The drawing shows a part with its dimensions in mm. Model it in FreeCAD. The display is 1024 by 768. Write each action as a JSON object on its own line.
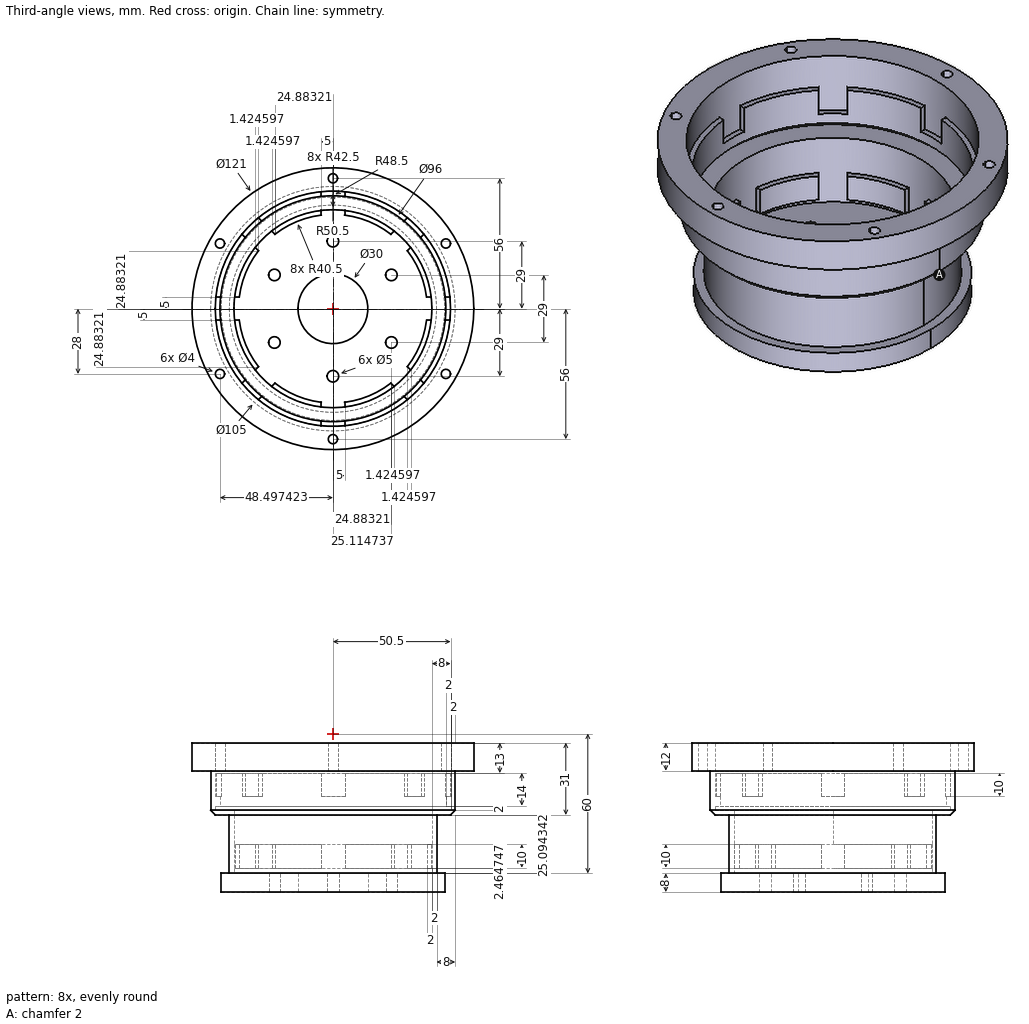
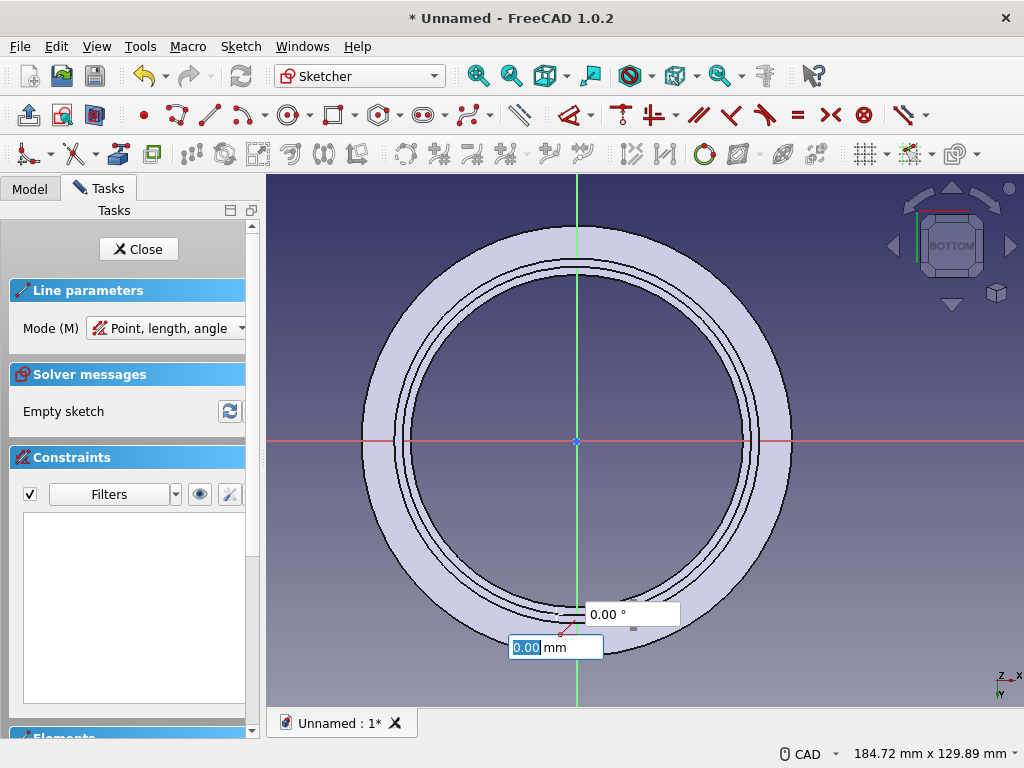
{"action": "scroll", "coordinate": [556, 606], "scroll_direction": "up", "scroll_amount": 4}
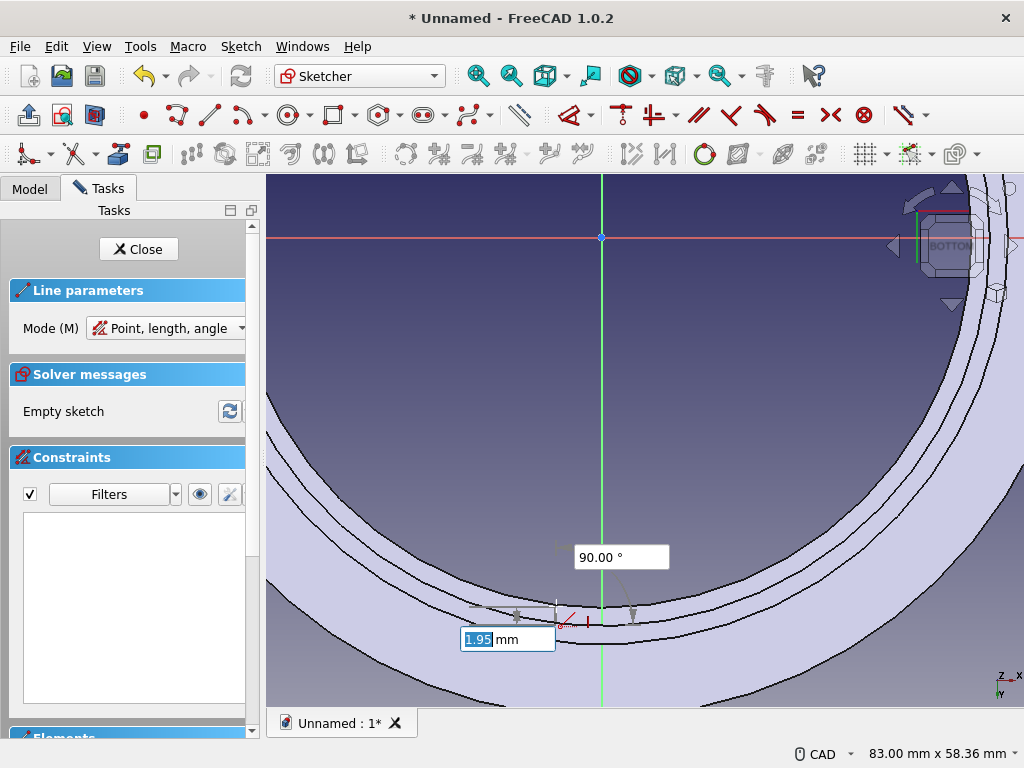
{"action": "left_click", "coordinate": [556, 605]}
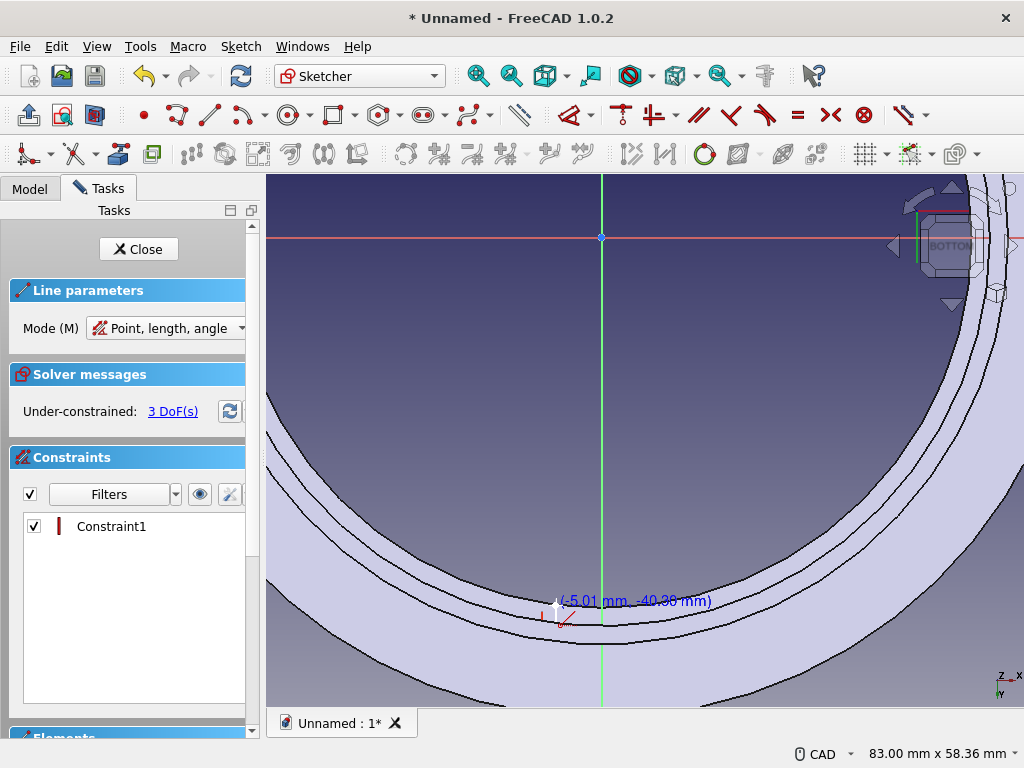
{"action": "left_click", "coordinate": [374, 530]}
{"action": "left_click", "coordinate": [361, 543]}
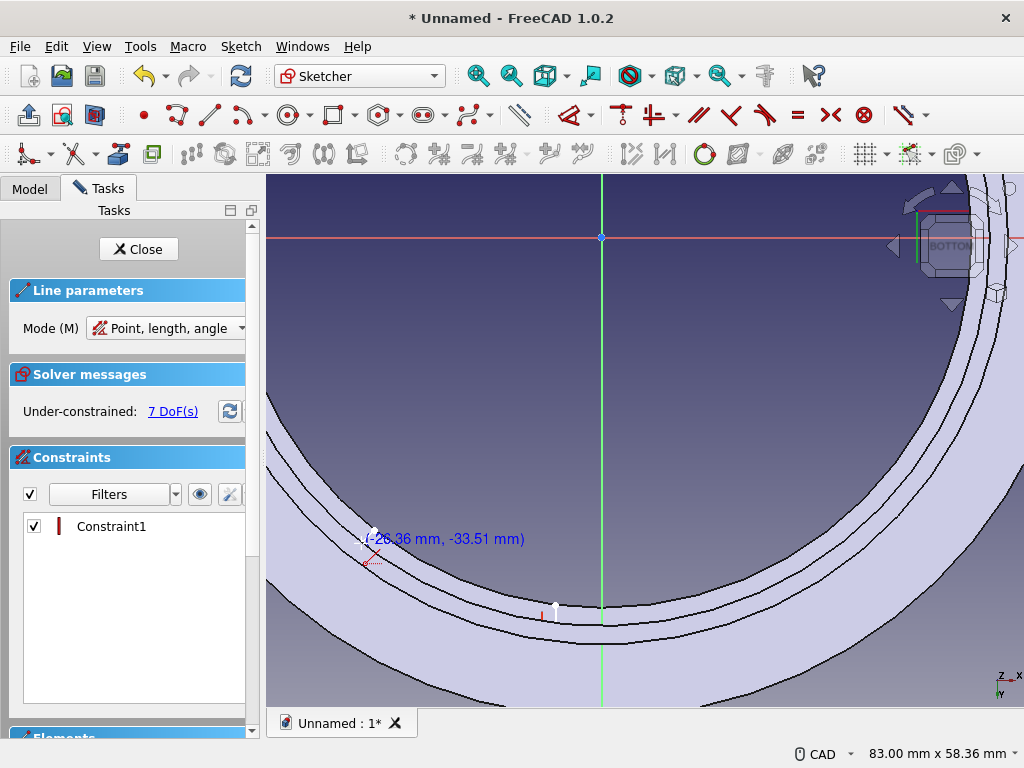
{"action": "left_click", "coordinate": [297, 478]}
{"action": "left_click", "coordinate": [310, 465]}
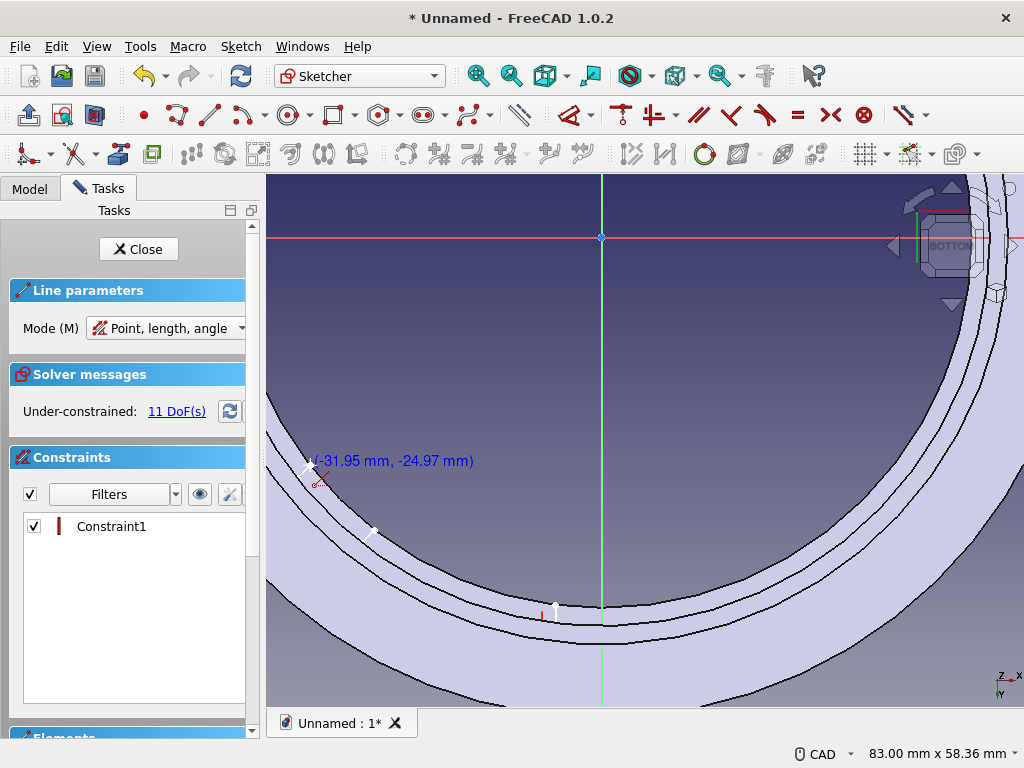
{"action": "scroll", "coordinate": [556, 606], "scroll_direction": "down", "scroll_amount": 4}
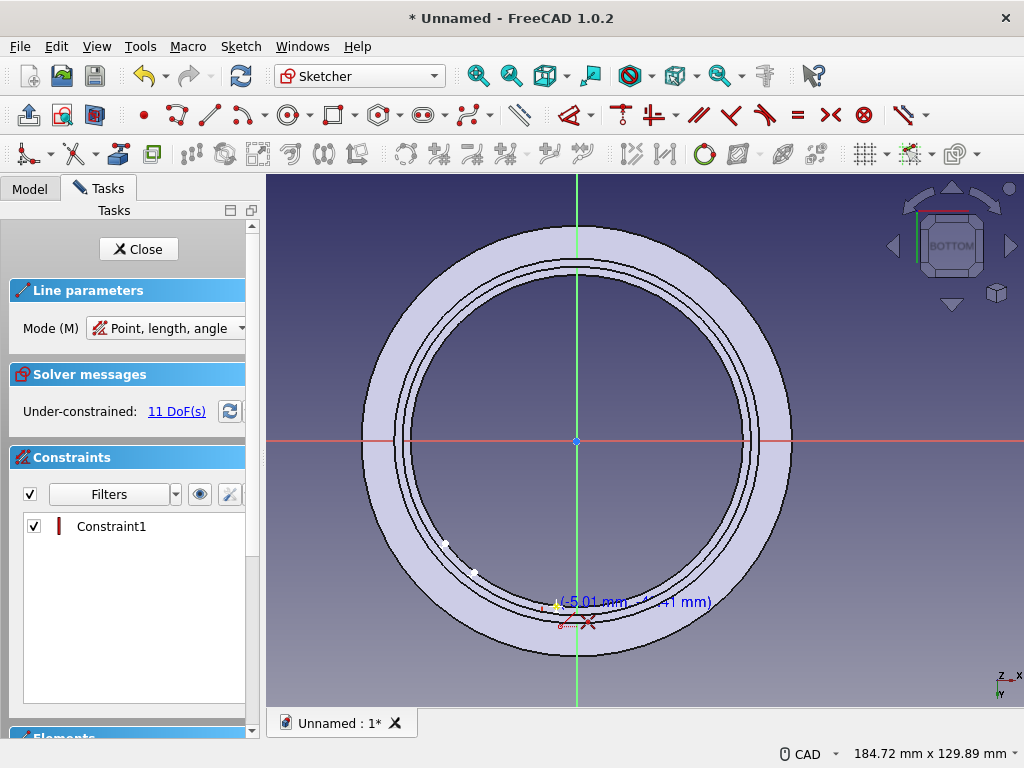
{"action": "left_click", "coordinate": [412, 462]}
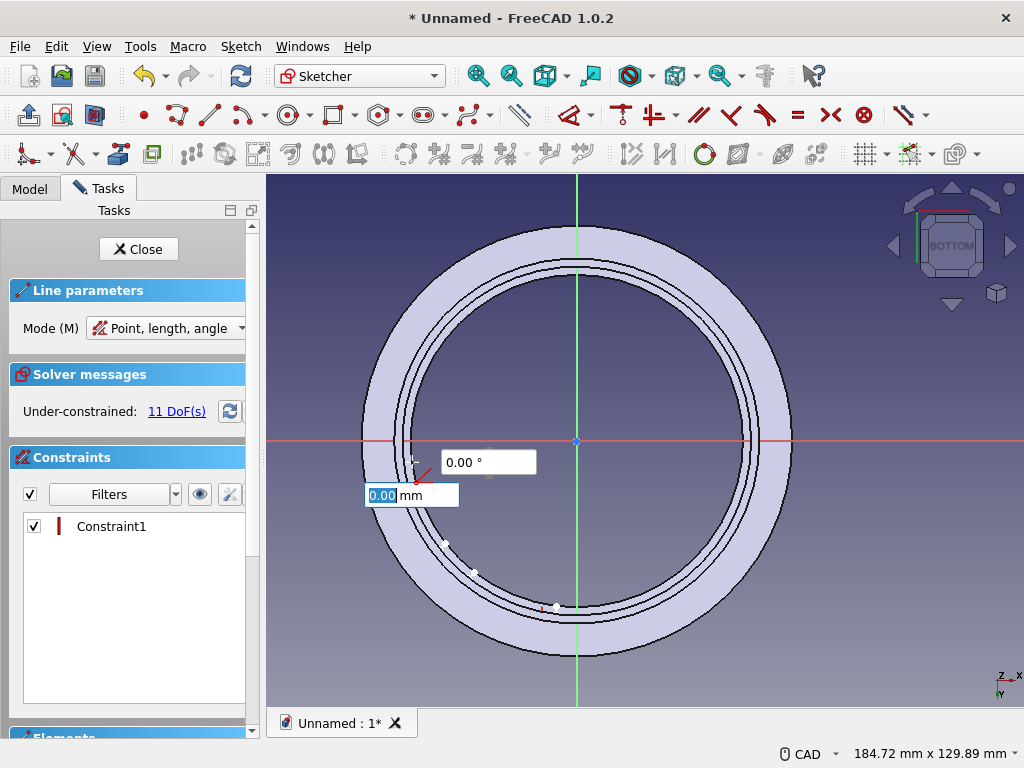
{"action": "scroll", "coordinate": [404, 462], "scroll_direction": "up", "scroll_amount": 4}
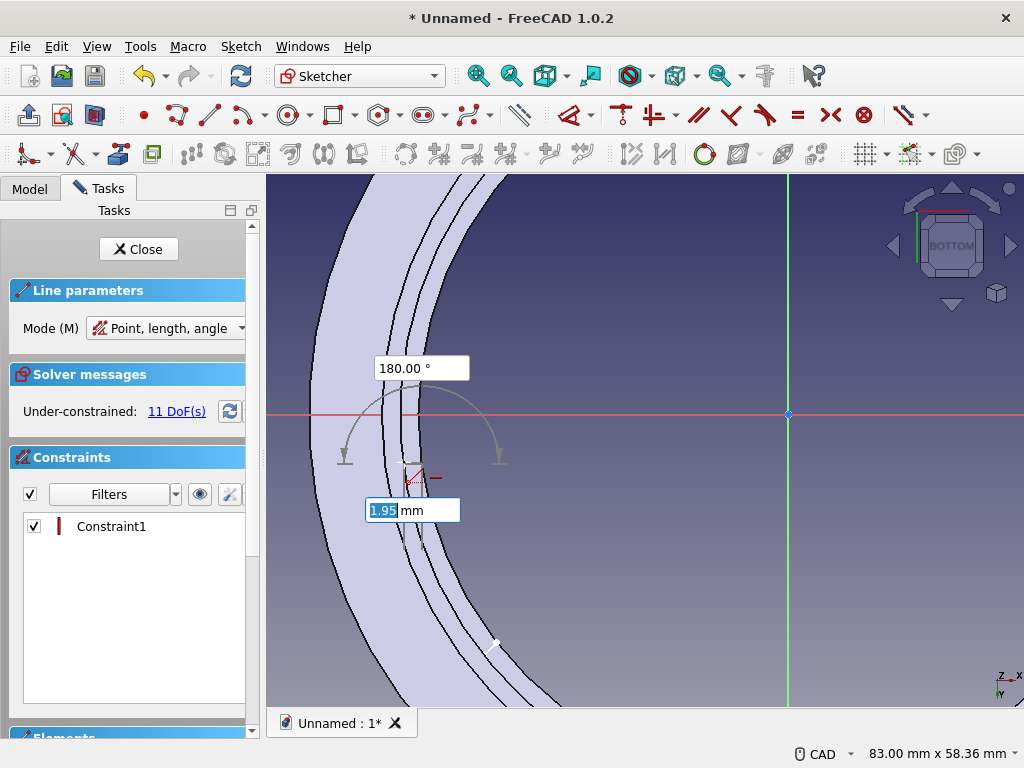
{"action": "left_click", "coordinate": [403, 461]}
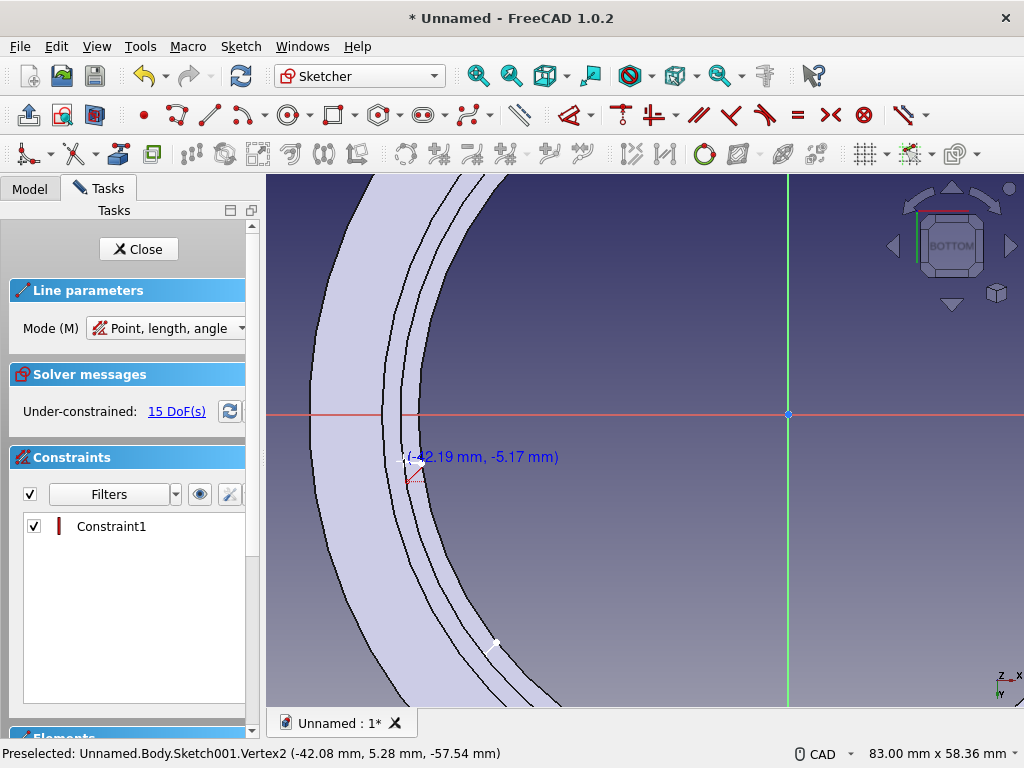
{"action": "left_click", "coordinate": [403, 369]}
{"action": "left_click", "coordinate": [421, 369]}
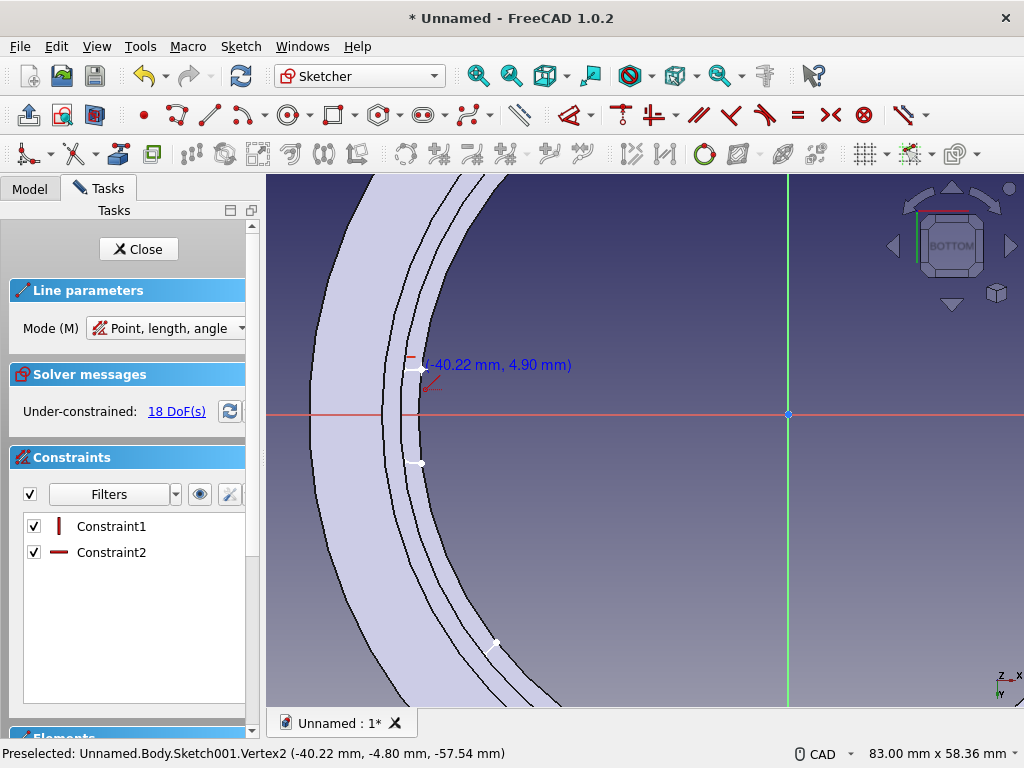
{"action": "scroll", "coordinate": [404, 462], "scroll_direction": "down", "scroll_amount": 4}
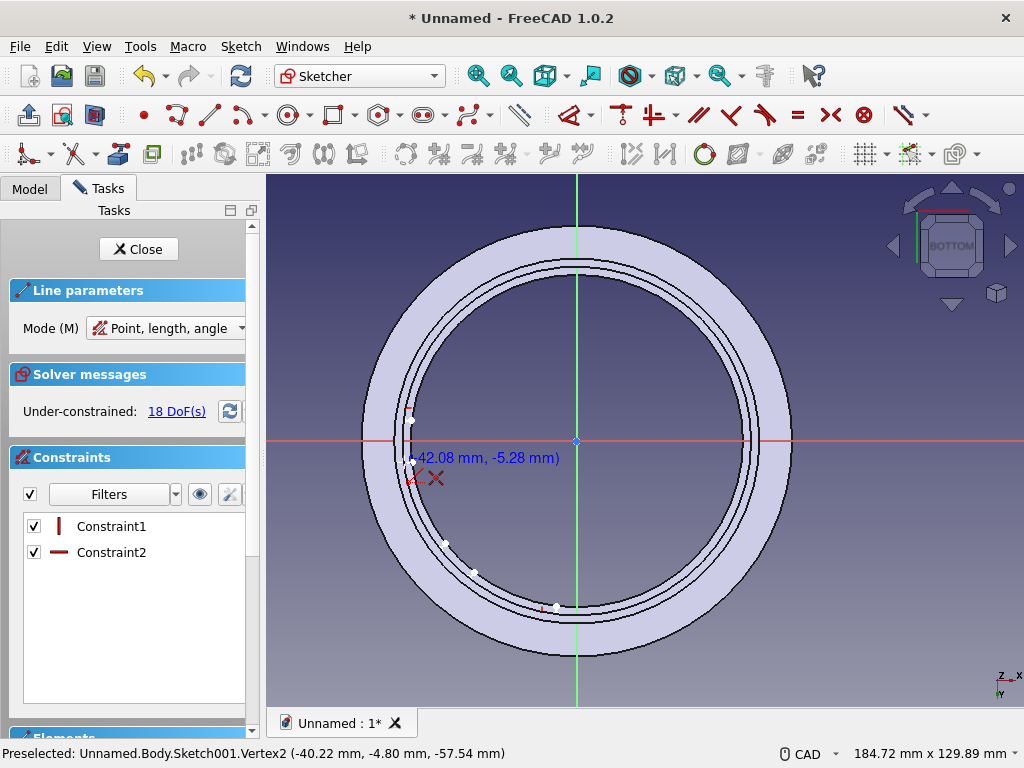
{"action": "left_click", "coordinate": [446, 339]}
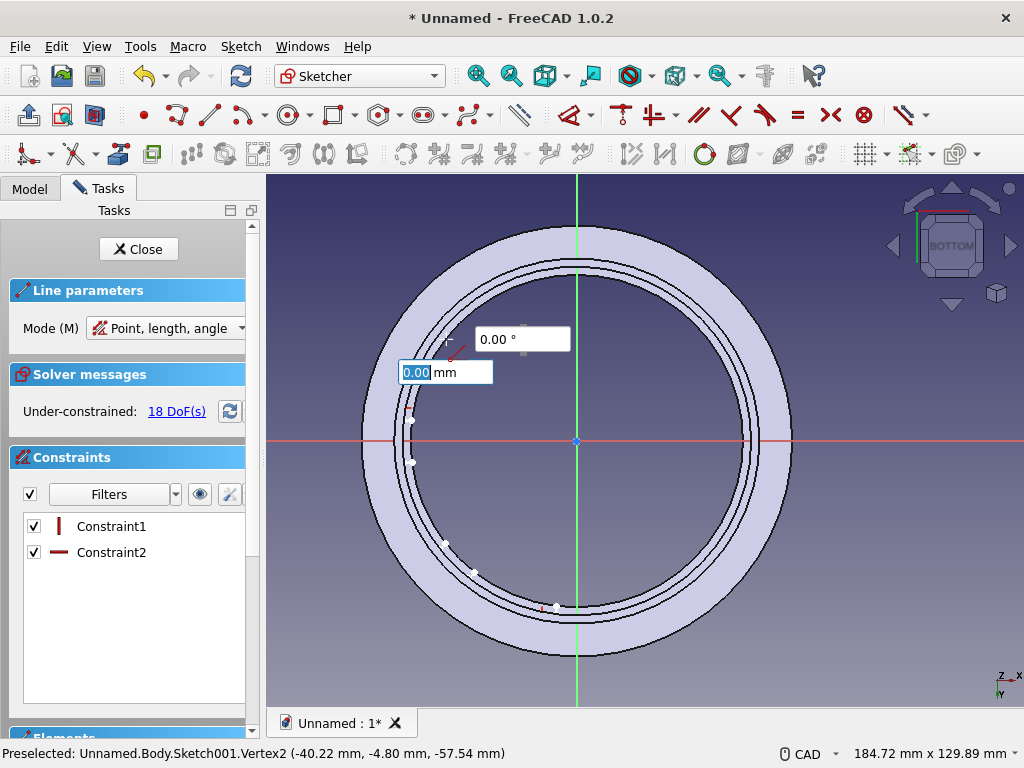
{"action": "scroll", "coordinate": [440, 333], "scroll_direction": "up", "scroll_amount": 4}